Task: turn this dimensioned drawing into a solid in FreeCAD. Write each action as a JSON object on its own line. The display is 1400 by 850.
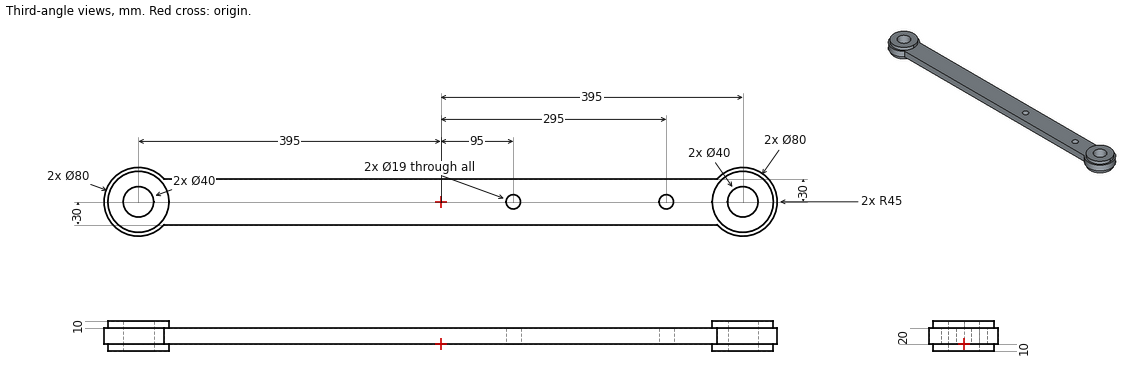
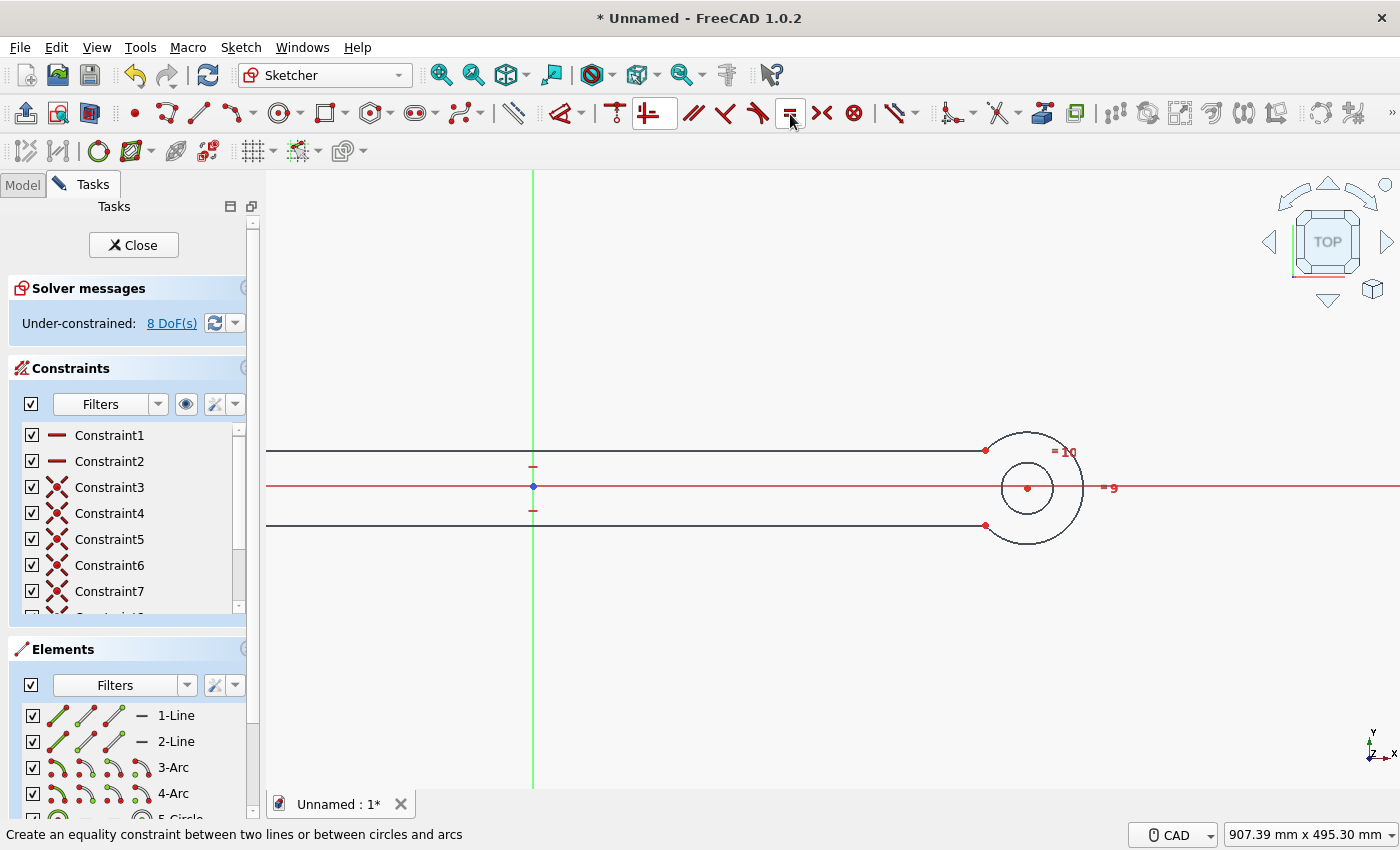
{"action": "scroll", "coordinate": [1045, 471], "scroll_direction": "down", "scroll_amount": 3}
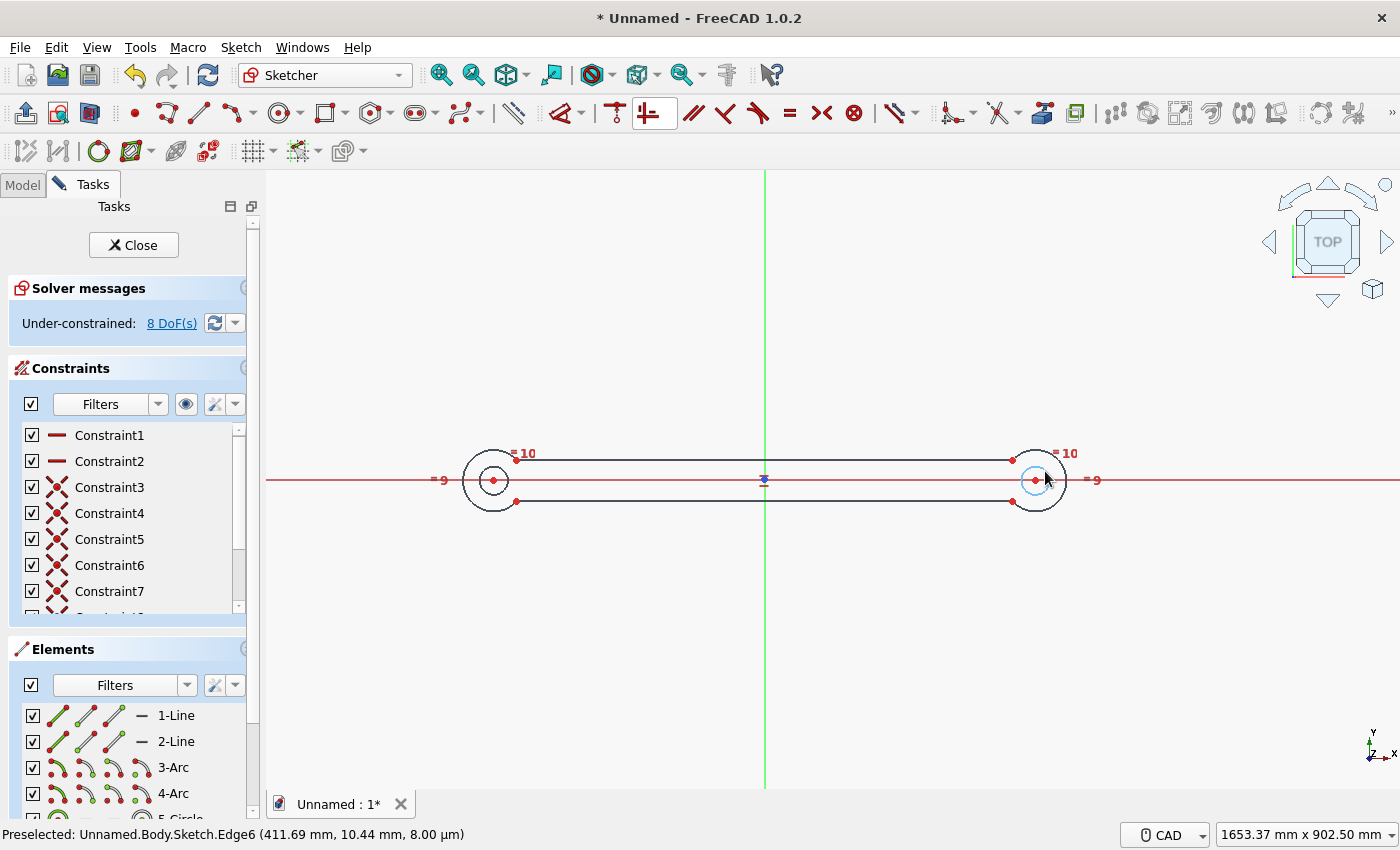
{"action": "left_click", "coordinate": [494, 481]}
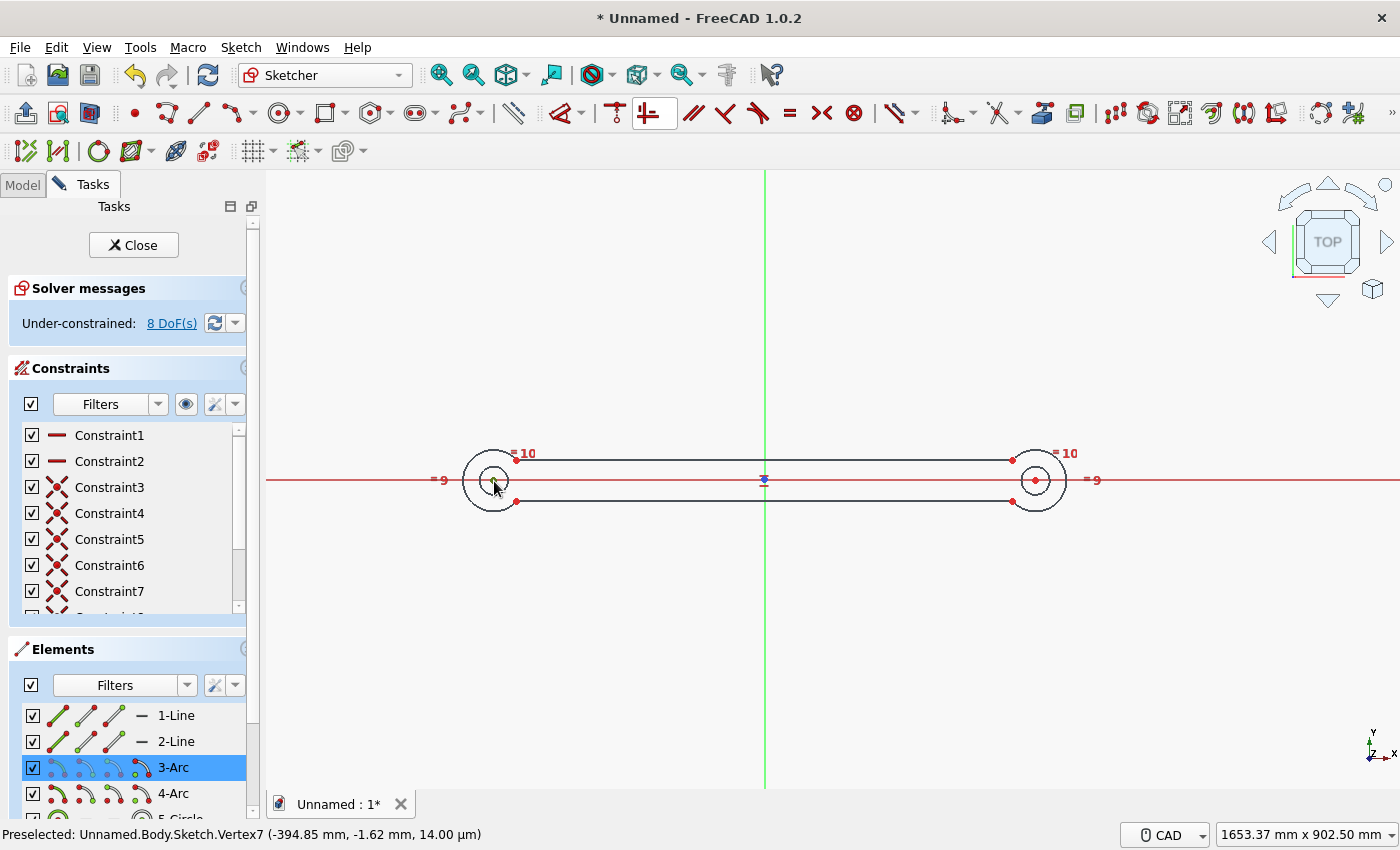
{"action": "left_click", "coordinate": [361, 480]}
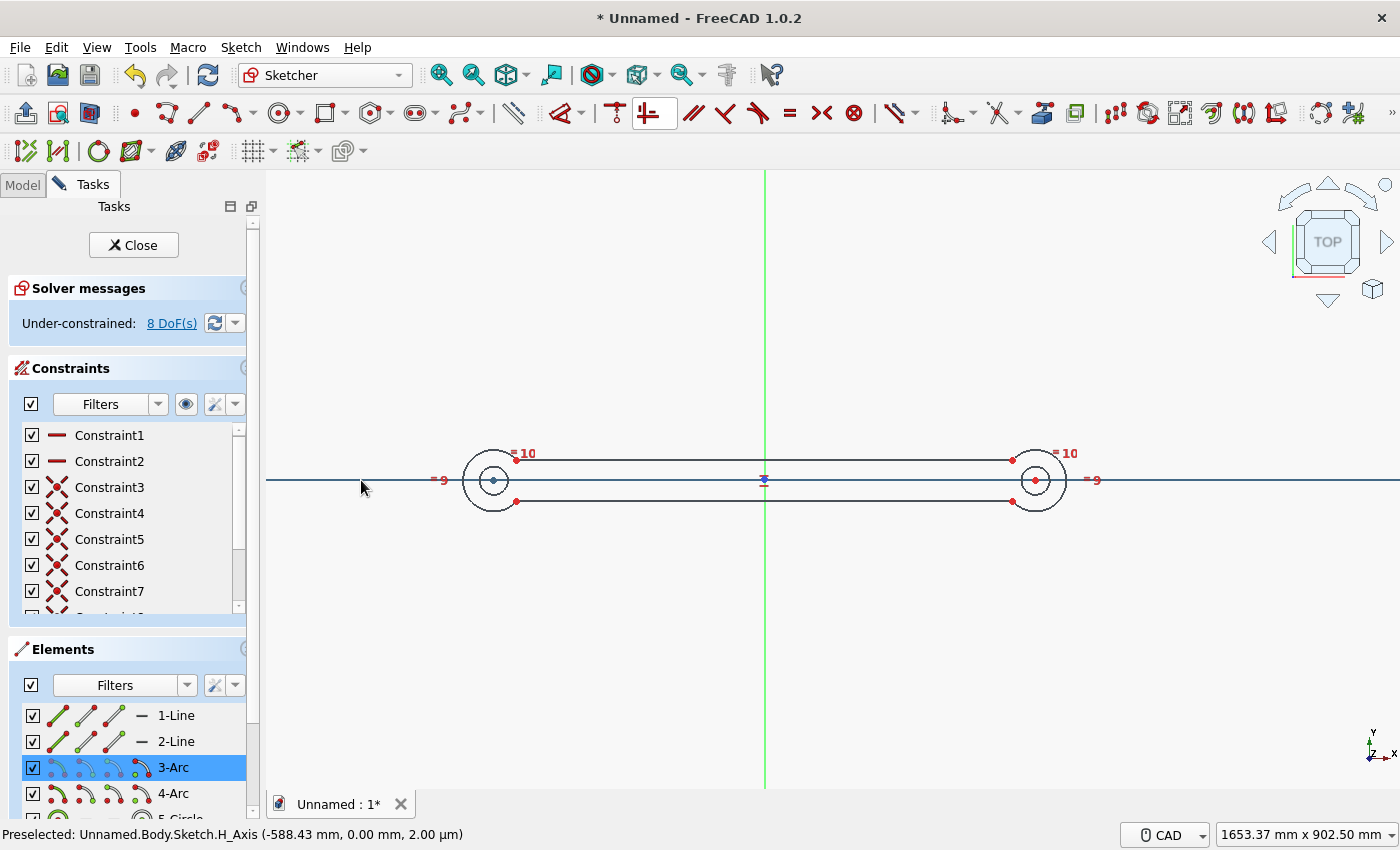
{"action": "left_click", "coordinate": [616, 114]}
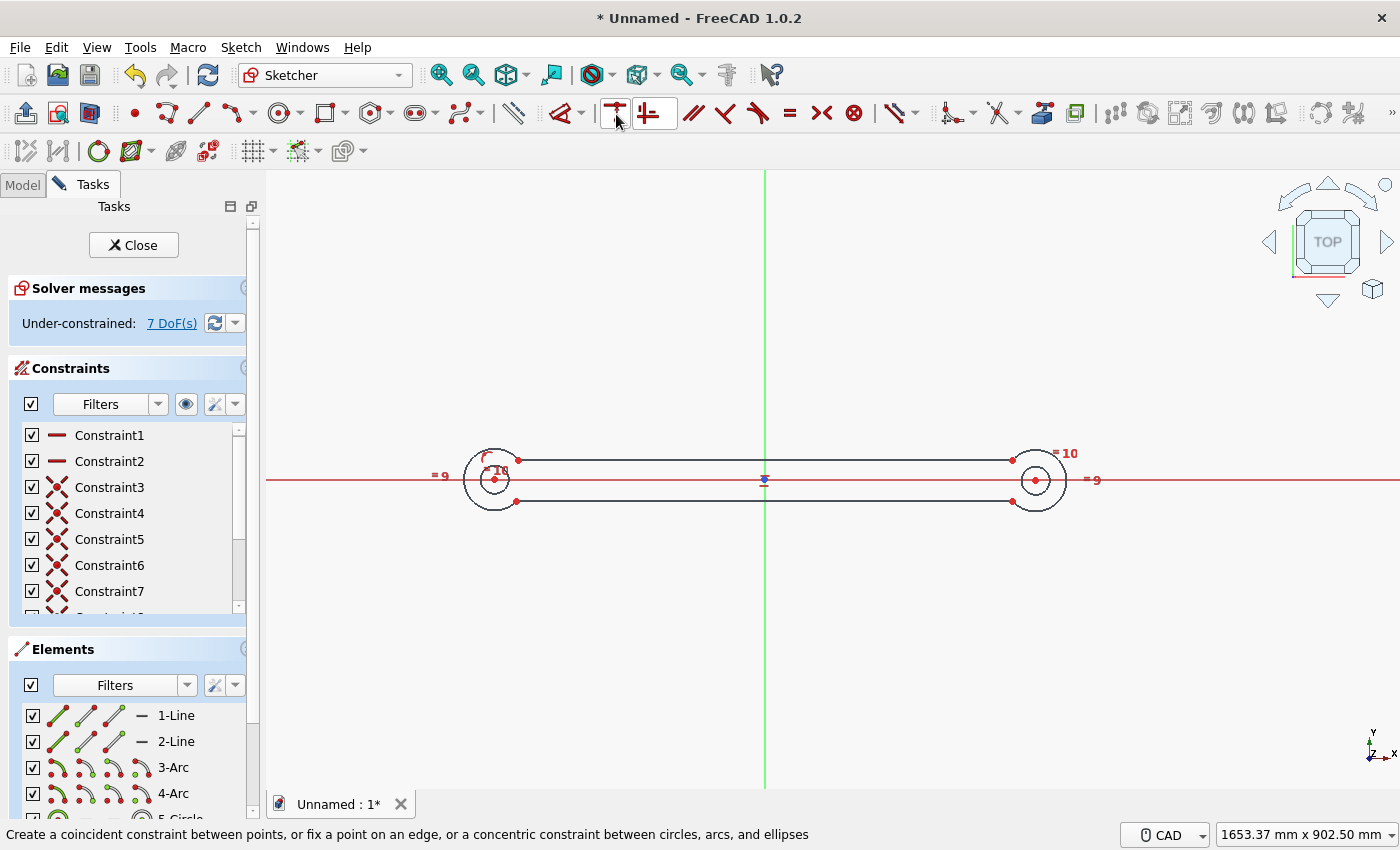
{"action": "left_click", "coordinate": [1036, 481]}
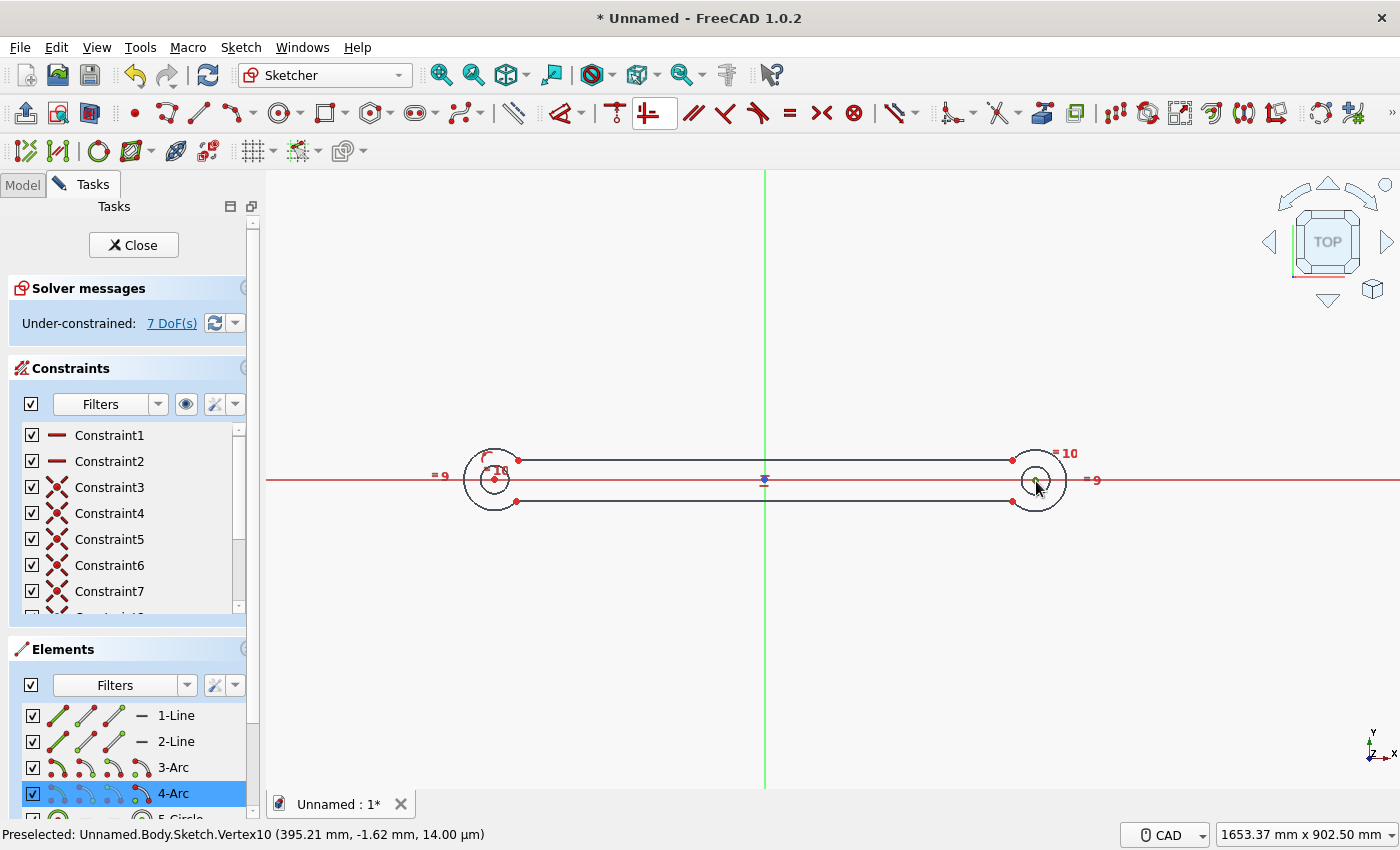
{"action": "left_click", "coordinate": [361, 480]}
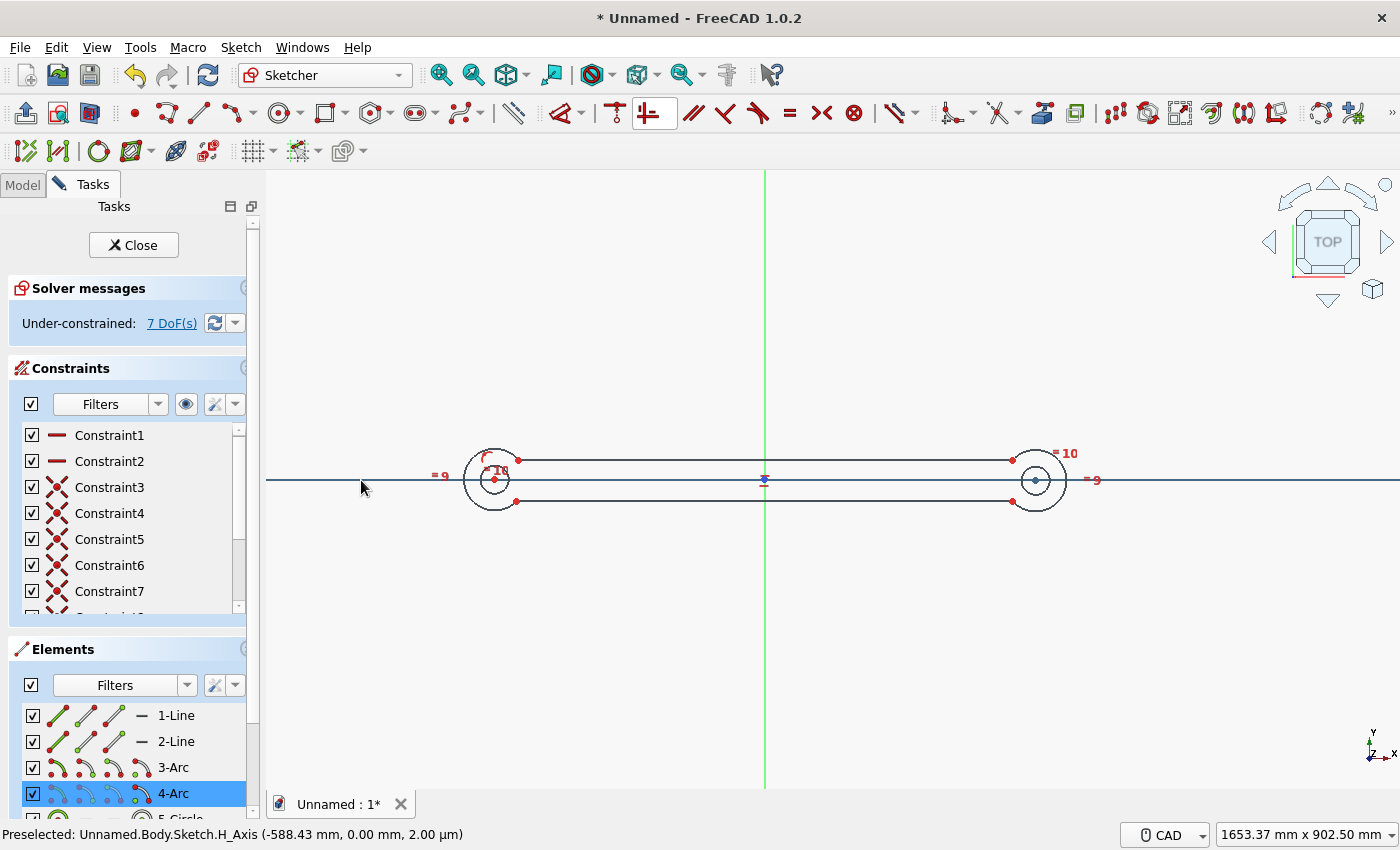
{"action": "left_click", "coordinate": [616, 114]}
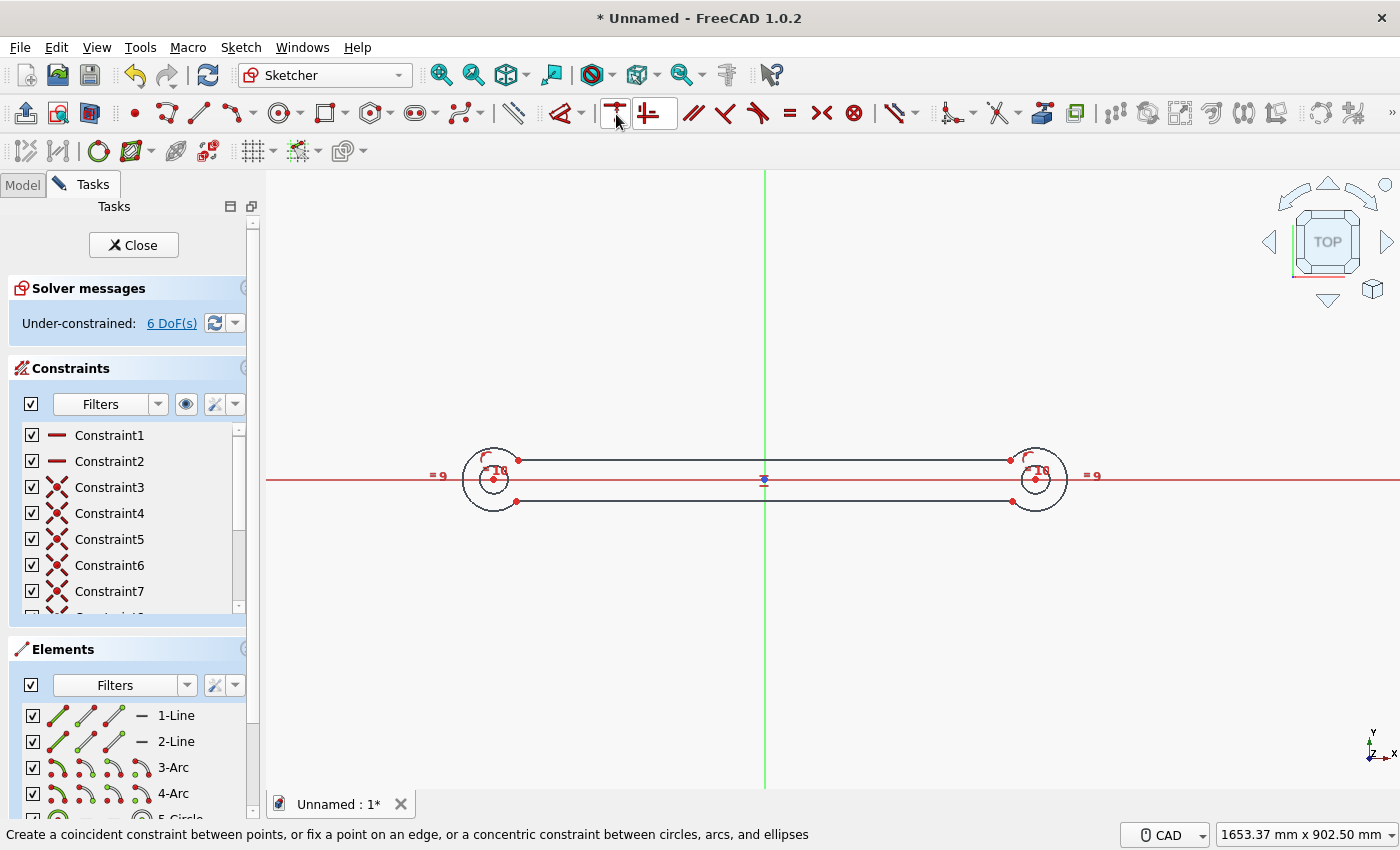
{"action": "left_click", "coordinate": [560, 114]}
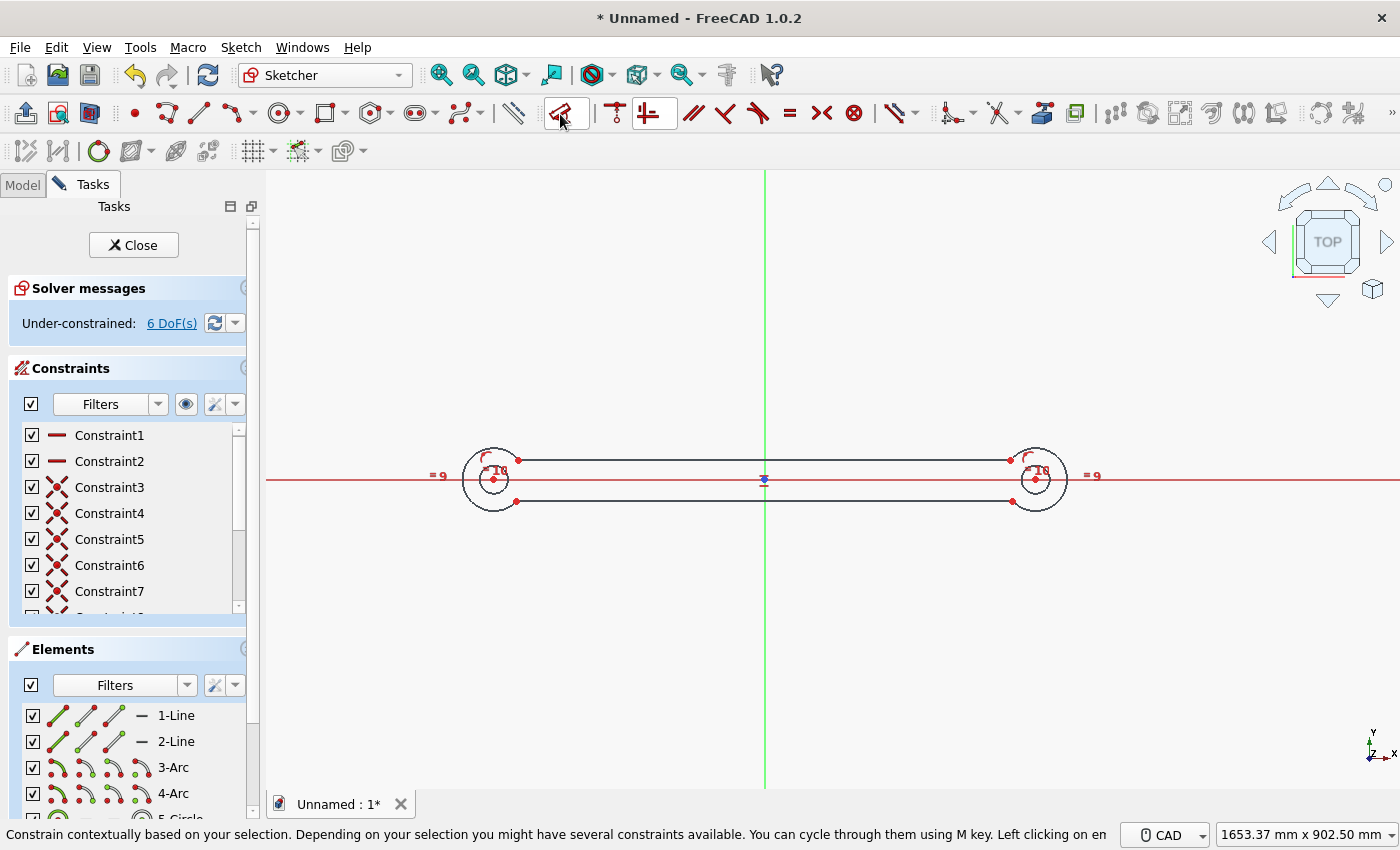
{"action": "scroll", "coordinate": [477, 453], "scroll_direction": "up", "scroll_amount": 2}